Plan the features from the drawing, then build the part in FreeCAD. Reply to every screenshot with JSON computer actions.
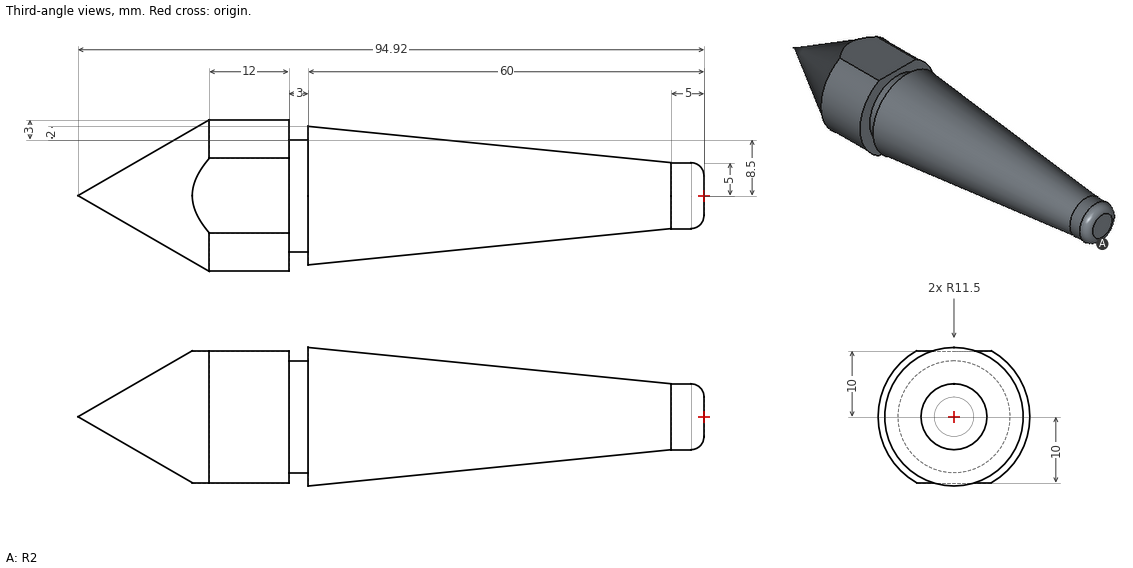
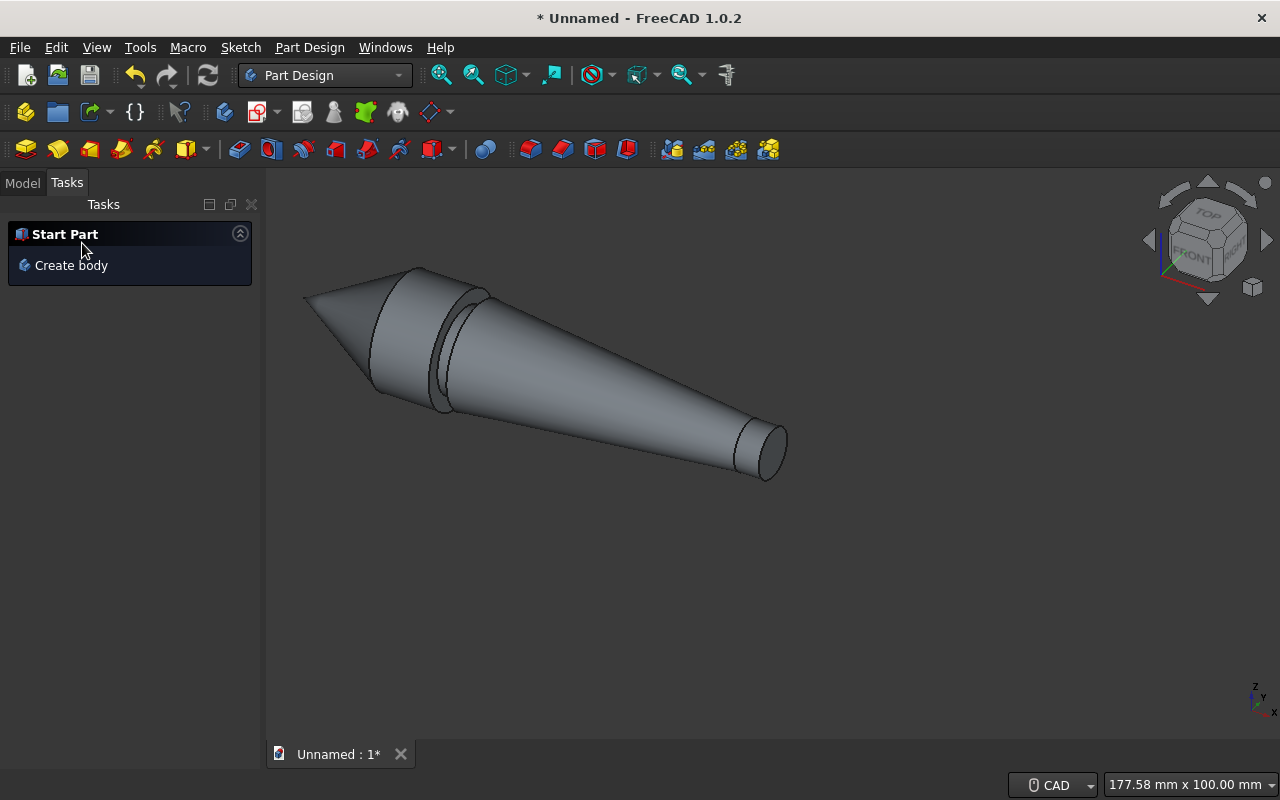
{"action": "left_click", "coordinate": [759, 467]}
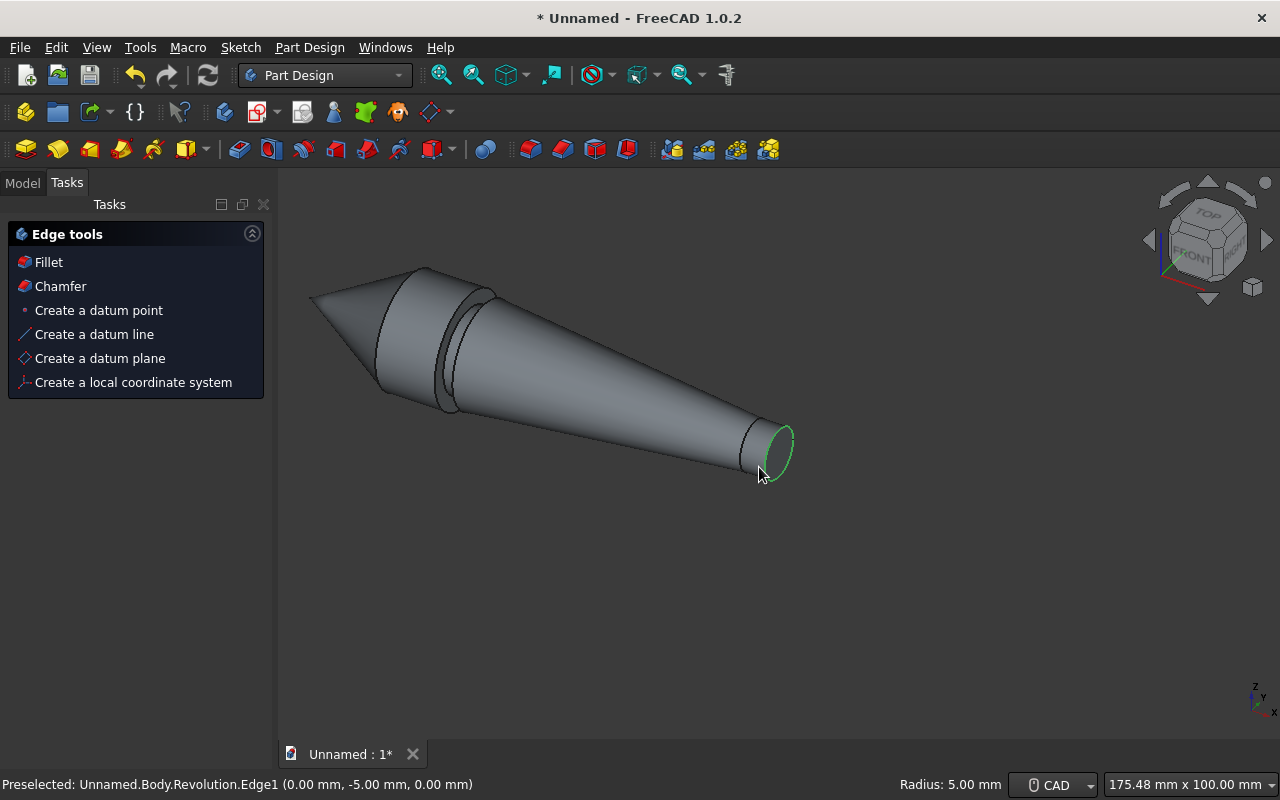
{"action": "left_click", "coordinate": [532, 150]}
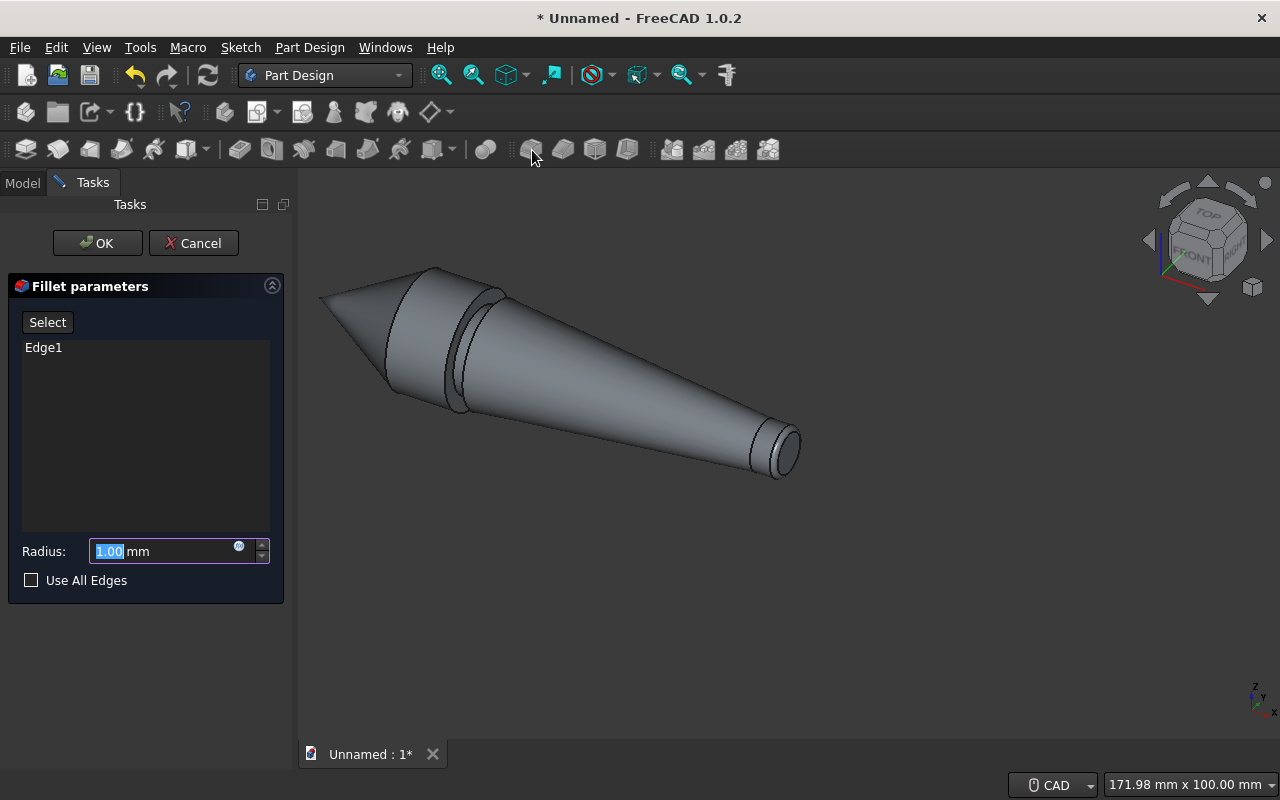
{"action": "type", "text": "2"}
{"action": "key", "text": "Tab"}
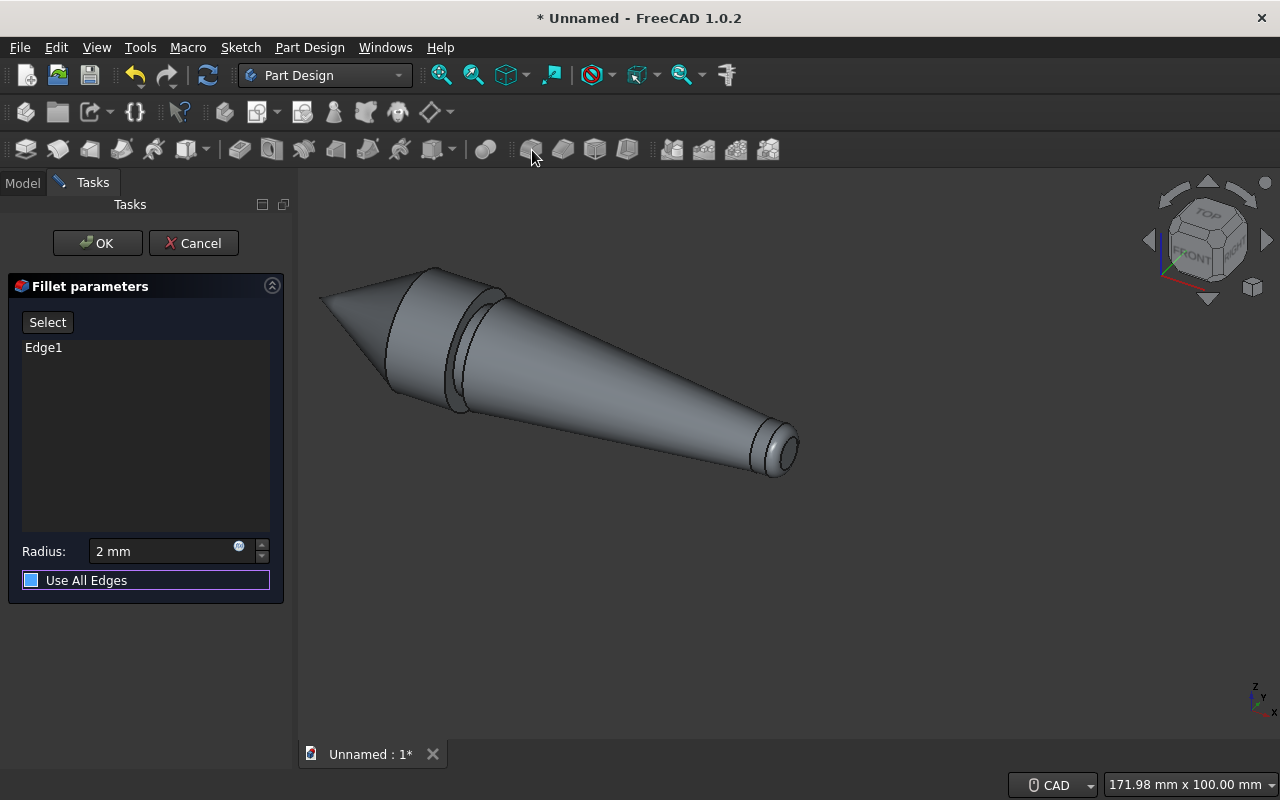
{"action": "left_click", "coordinate": [98, 243]}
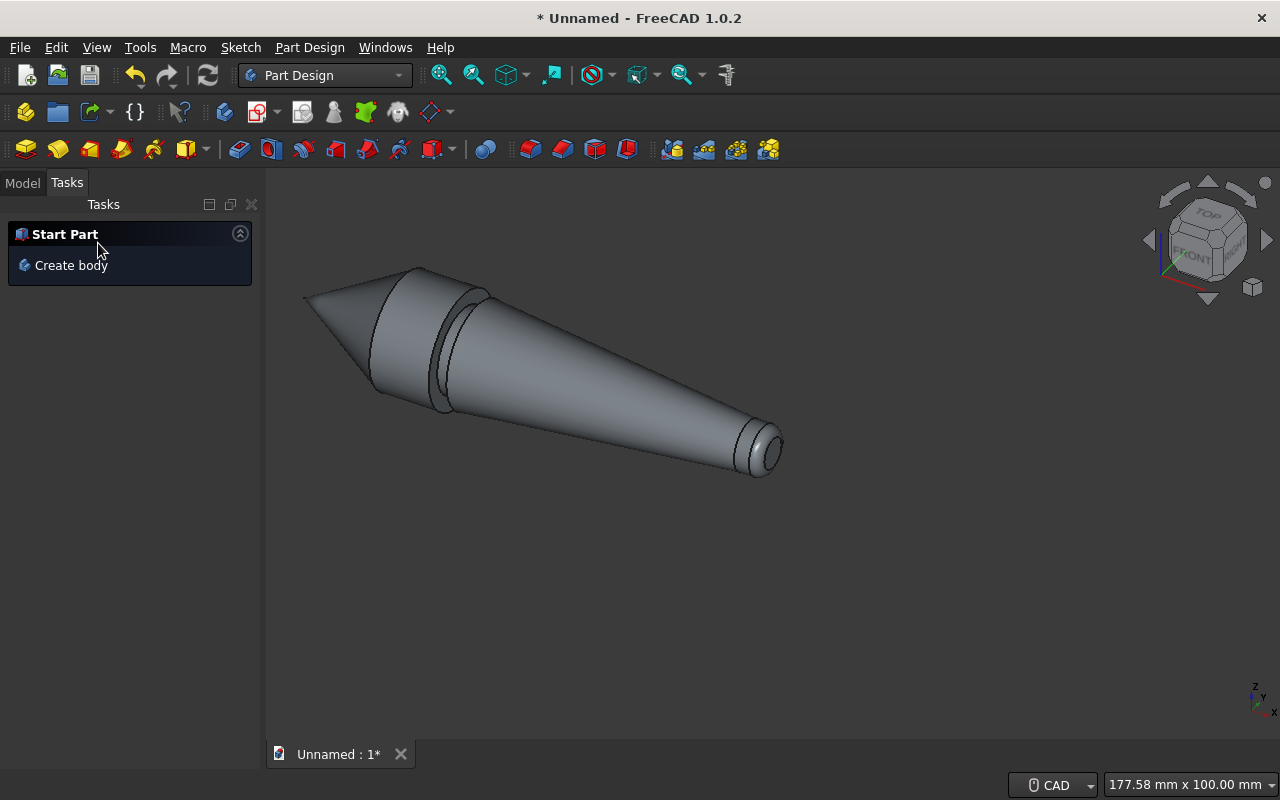
{"action": "left_click", "coordinate": [23, 182]}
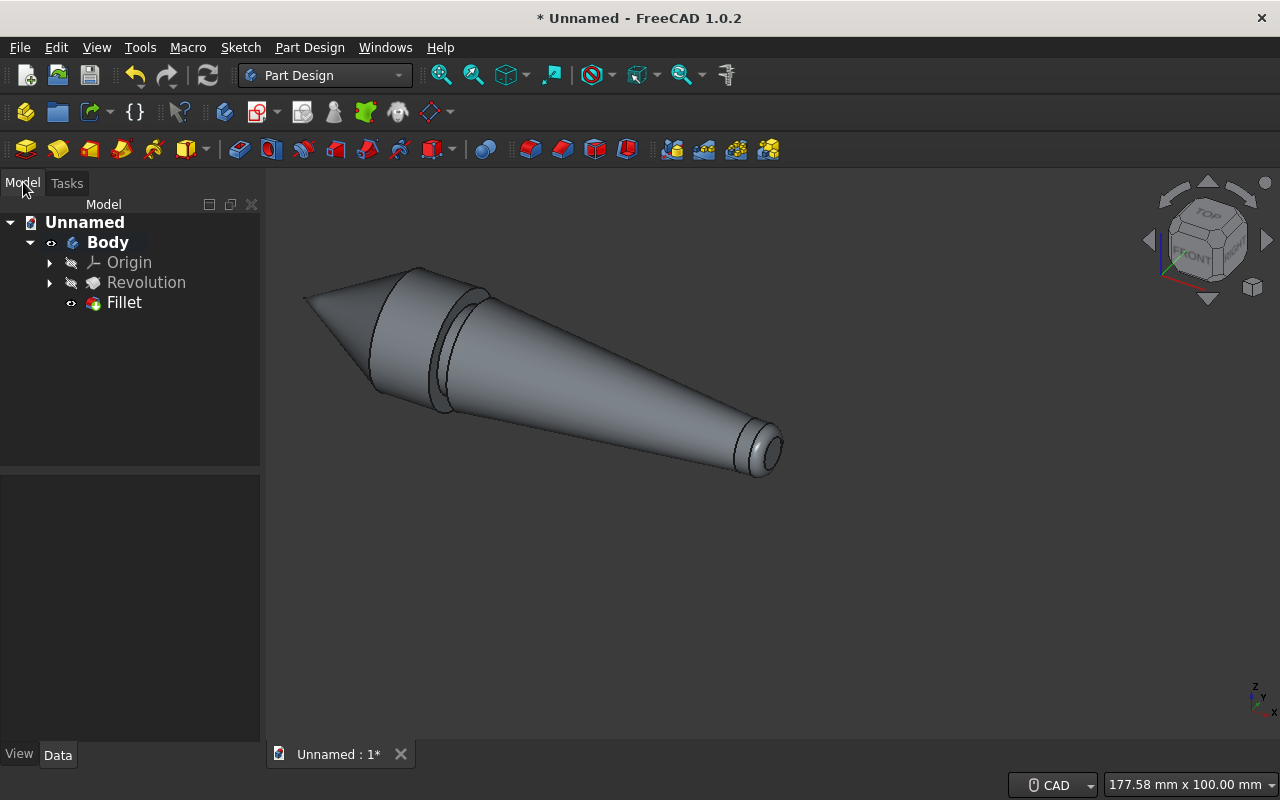
{"action": "left_click", "coordinate": [50, 263]}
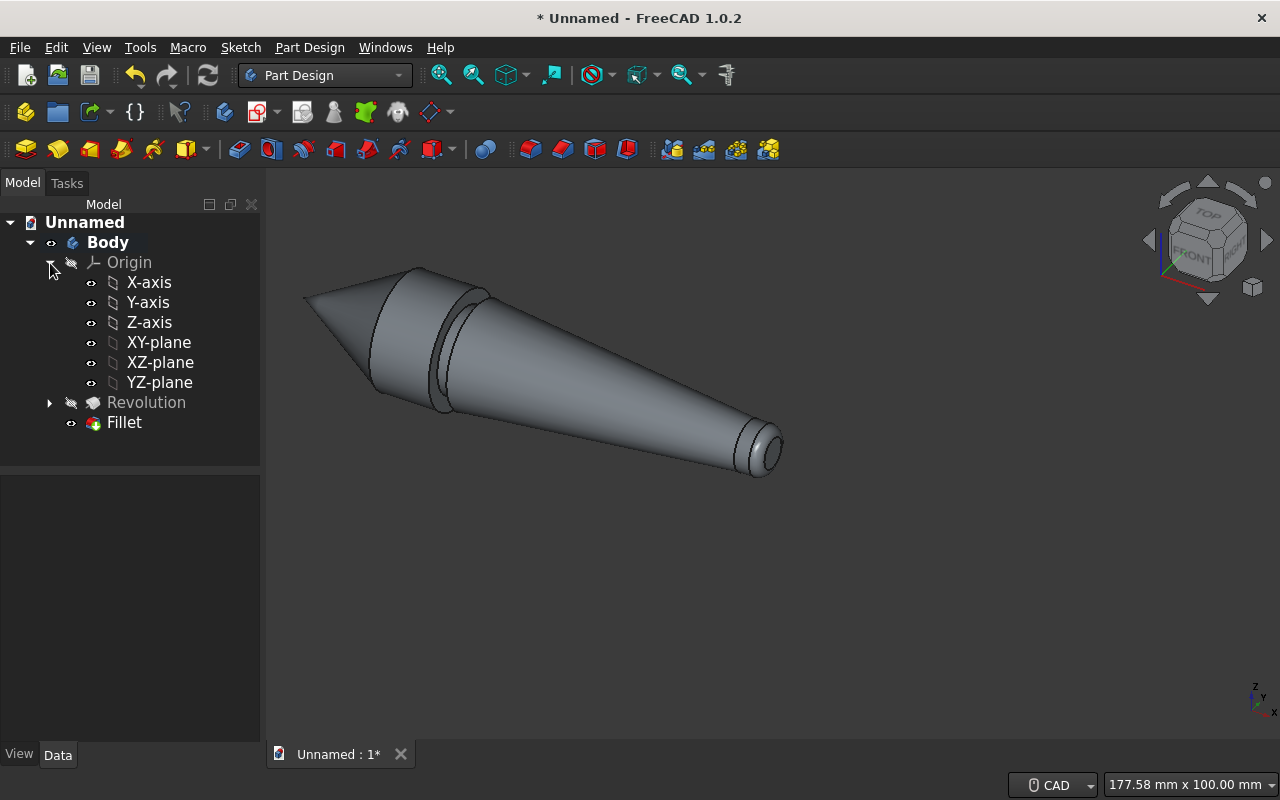
{"action": "left_click", "coordinate": [136, 383]}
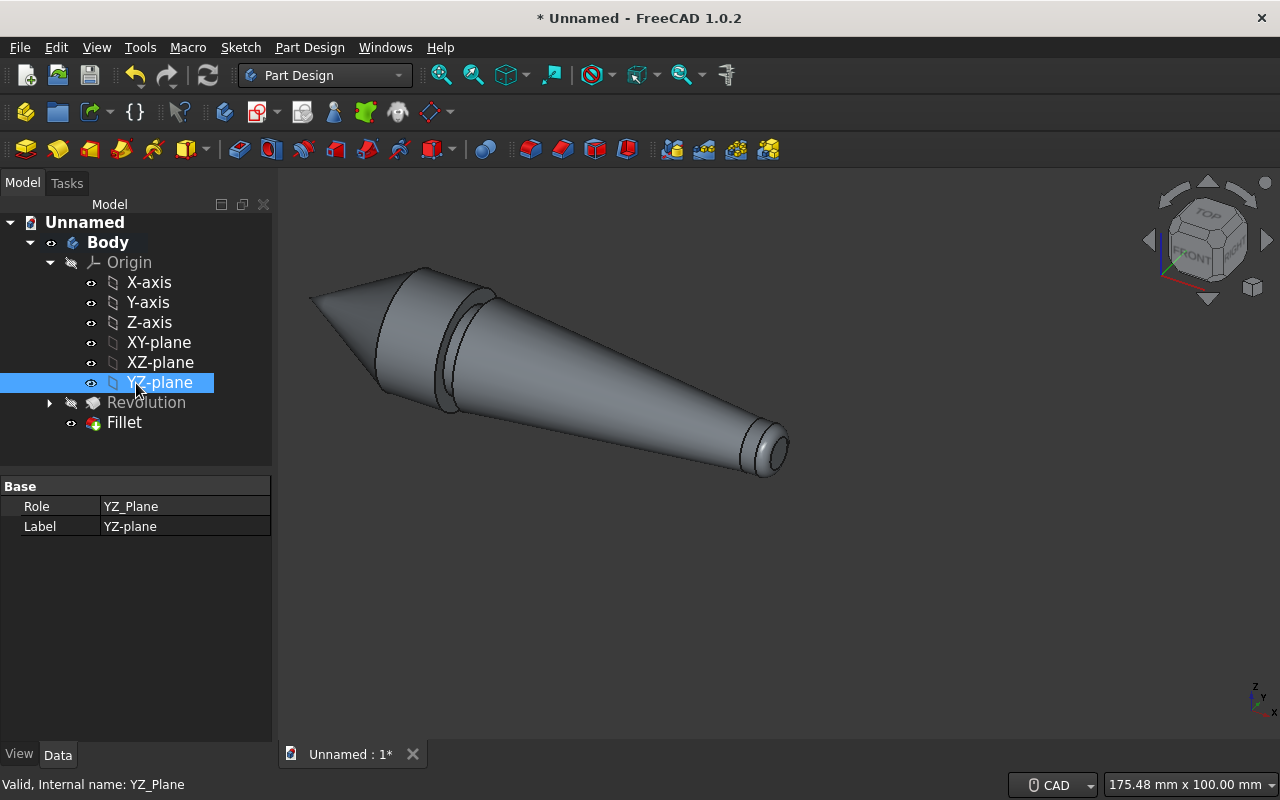
{"action": "left_click", "coordinate": [430, 112]}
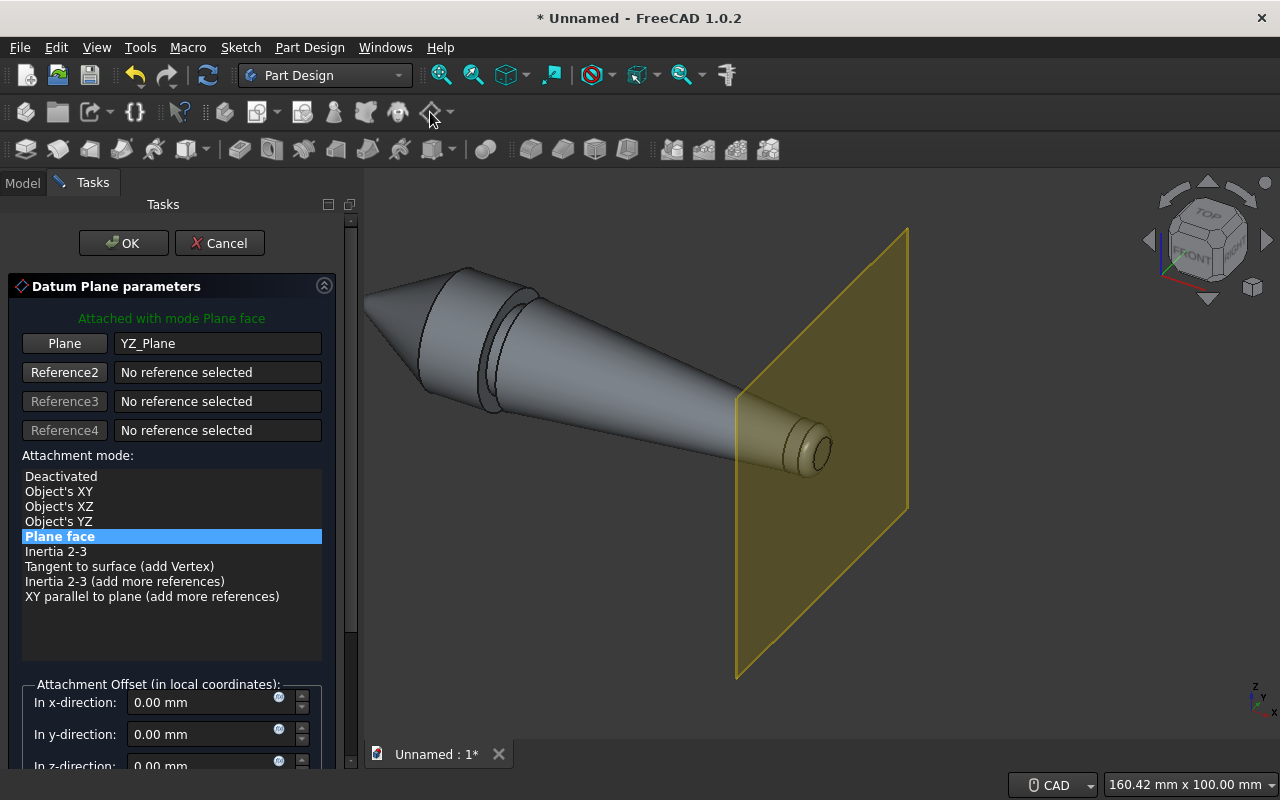
{"action": "scroll", "coordinate": [351, 491], "scroll_direction": "down", "scroll_amount": 2}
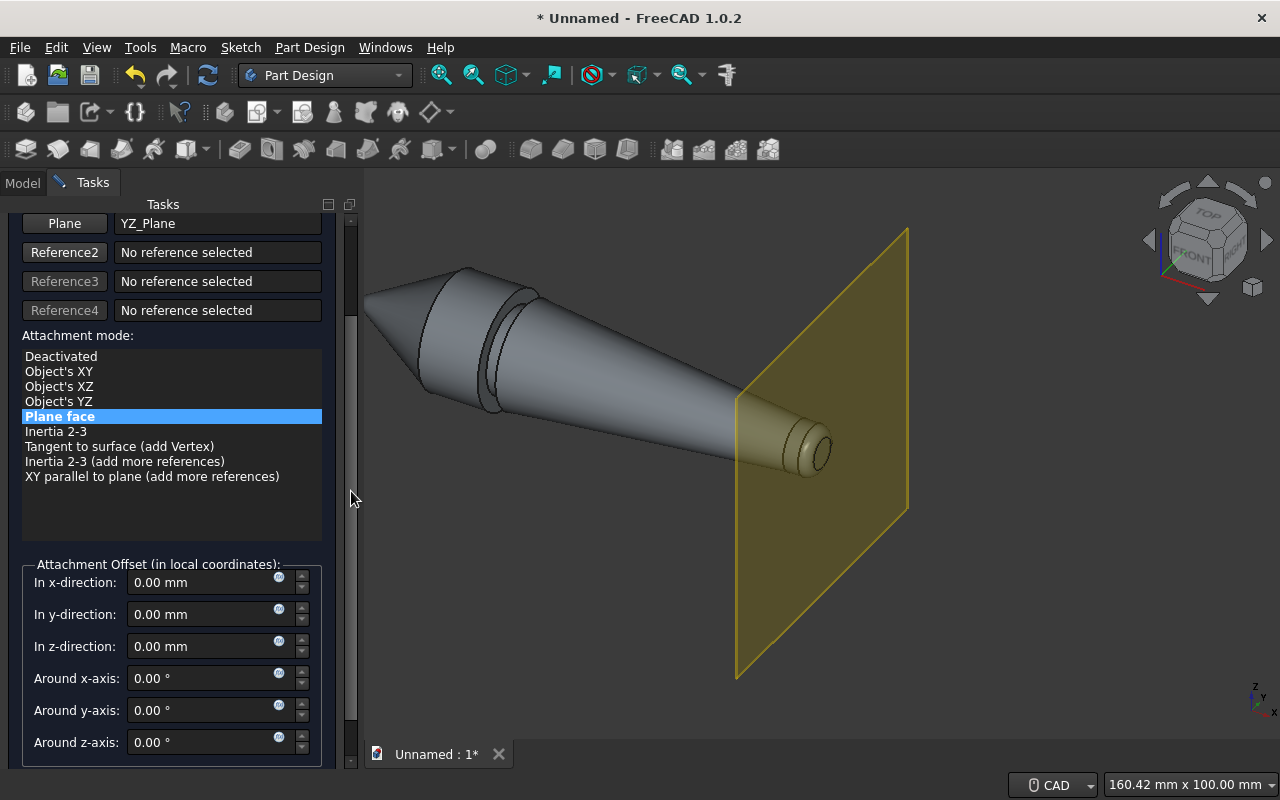
{"action": "triple_click", "coordinate": [210, 646]}